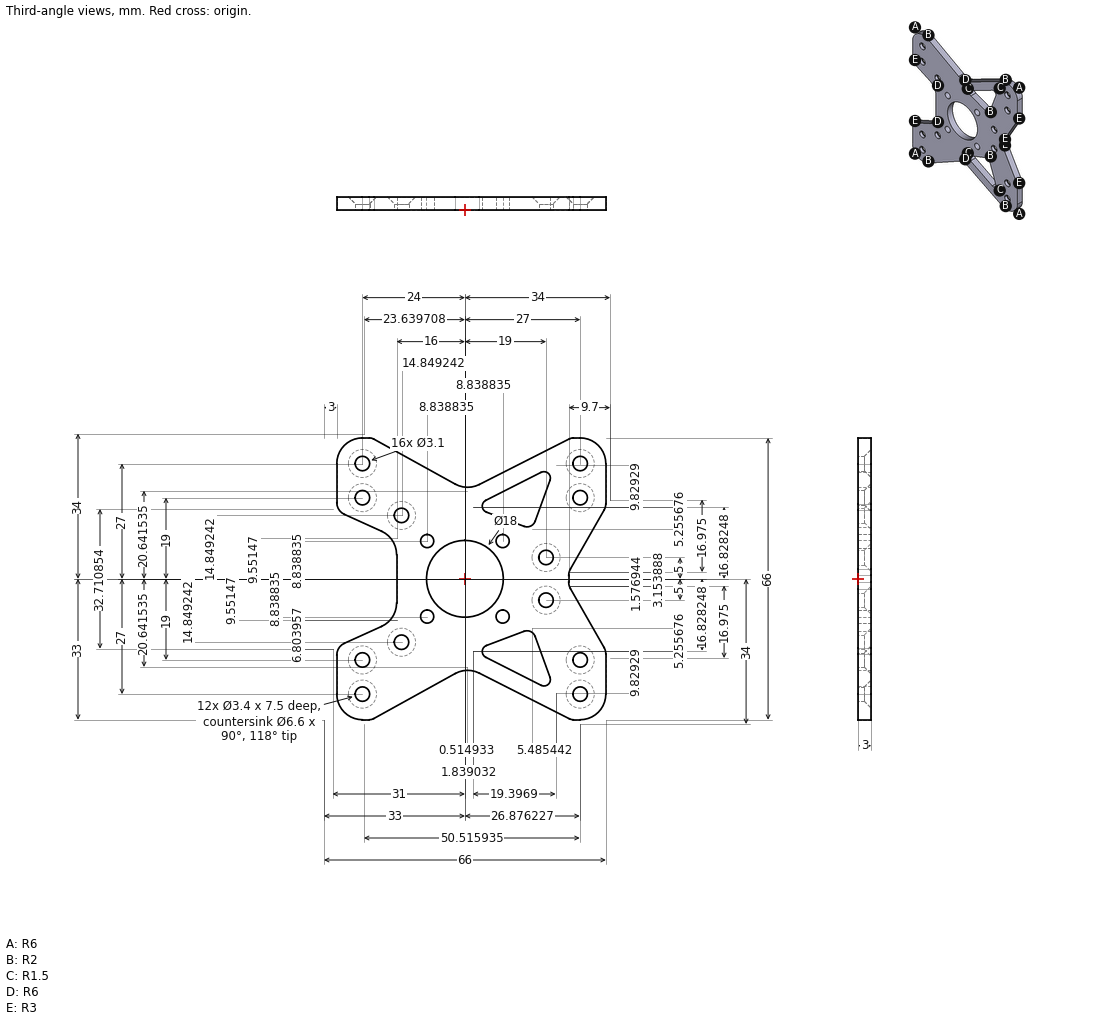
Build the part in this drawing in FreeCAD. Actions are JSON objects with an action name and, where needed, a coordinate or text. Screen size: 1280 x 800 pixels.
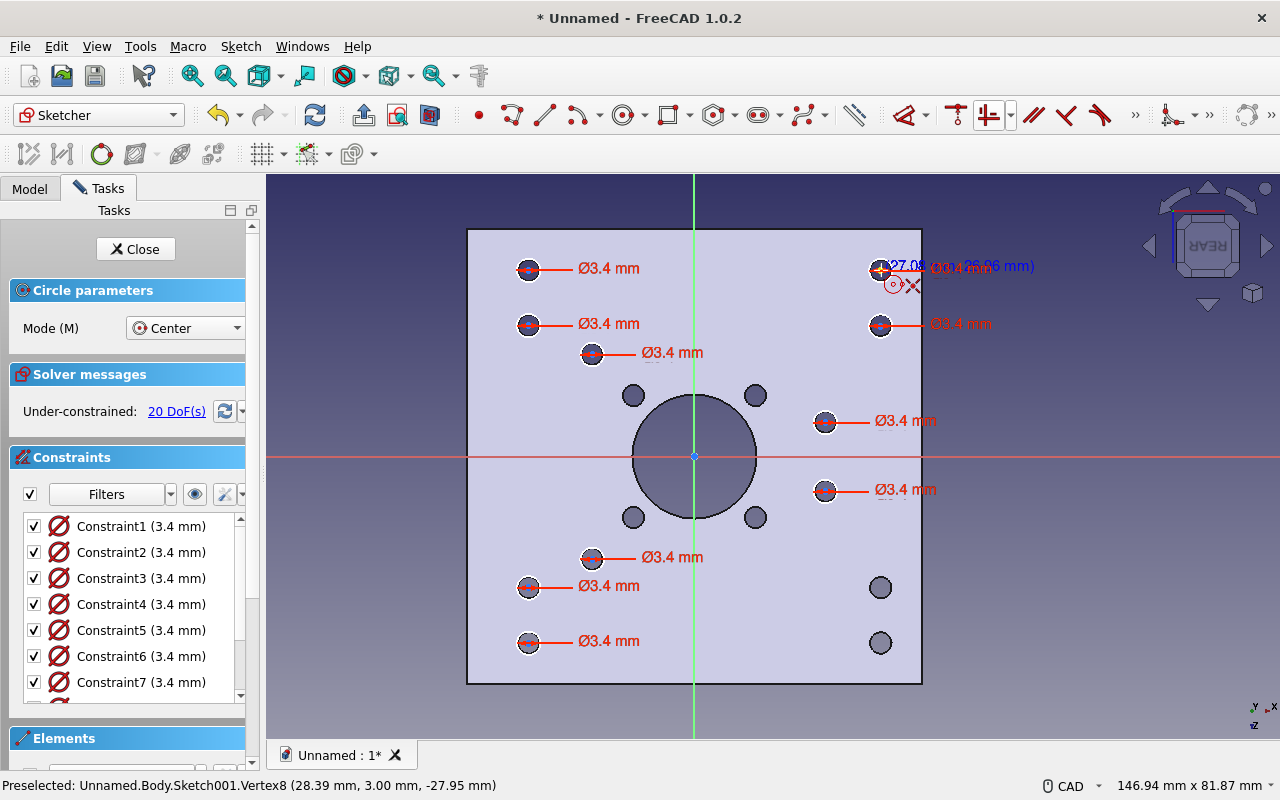
{"action": "scroll", "coordinate": [881, 588], "scroll_direction": "up", "scroll_amount": 4}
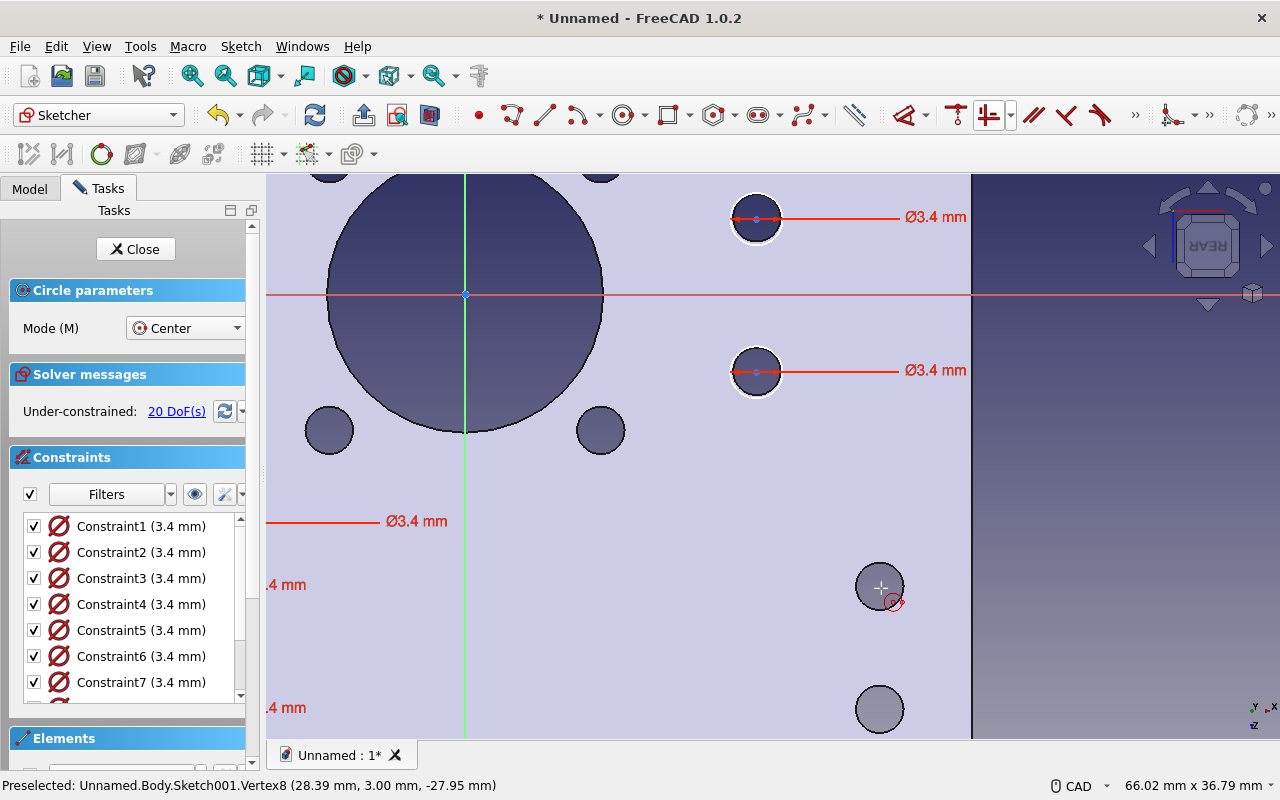
{"action": "left_click", "coordinate": [880, 586]}
{"action": "mouse_move", "coordinate": [898, 568]}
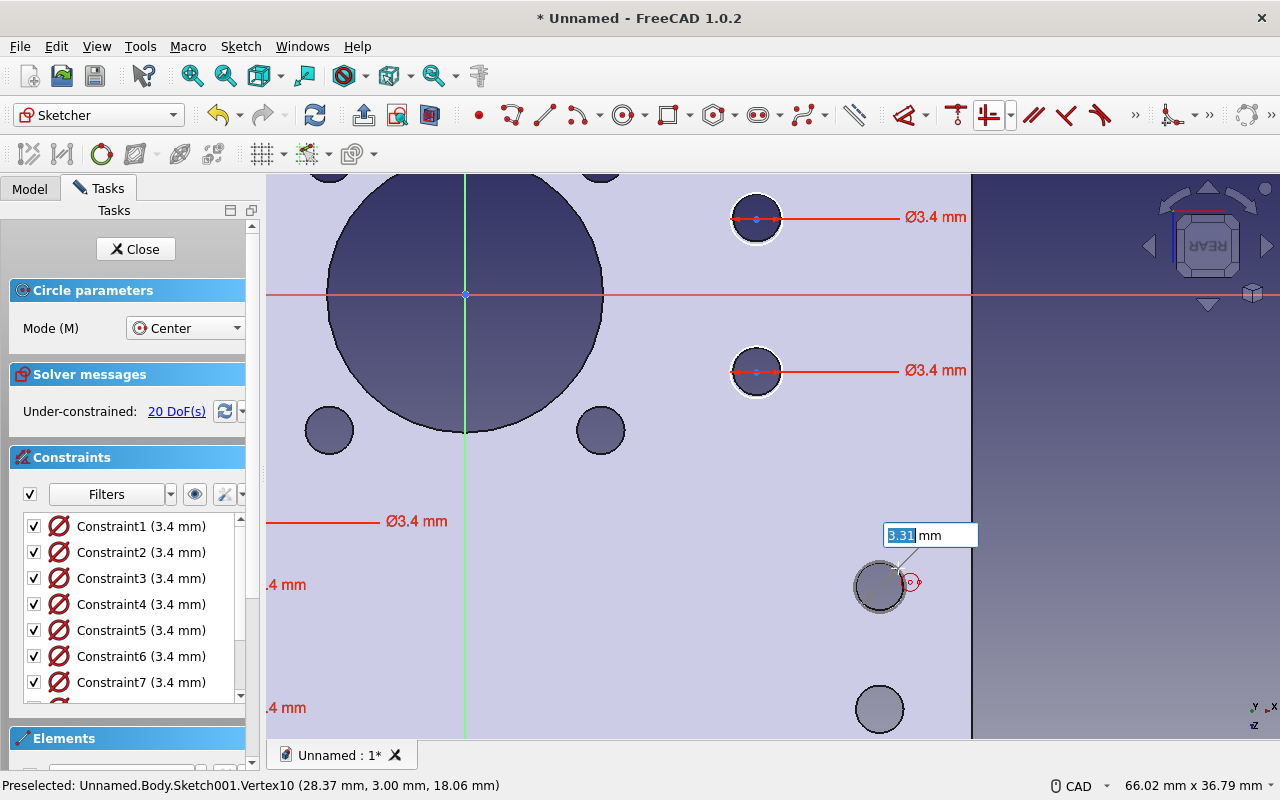
{"action": "type", "text": "3.4"}
{"action": "key", "text": "Return"}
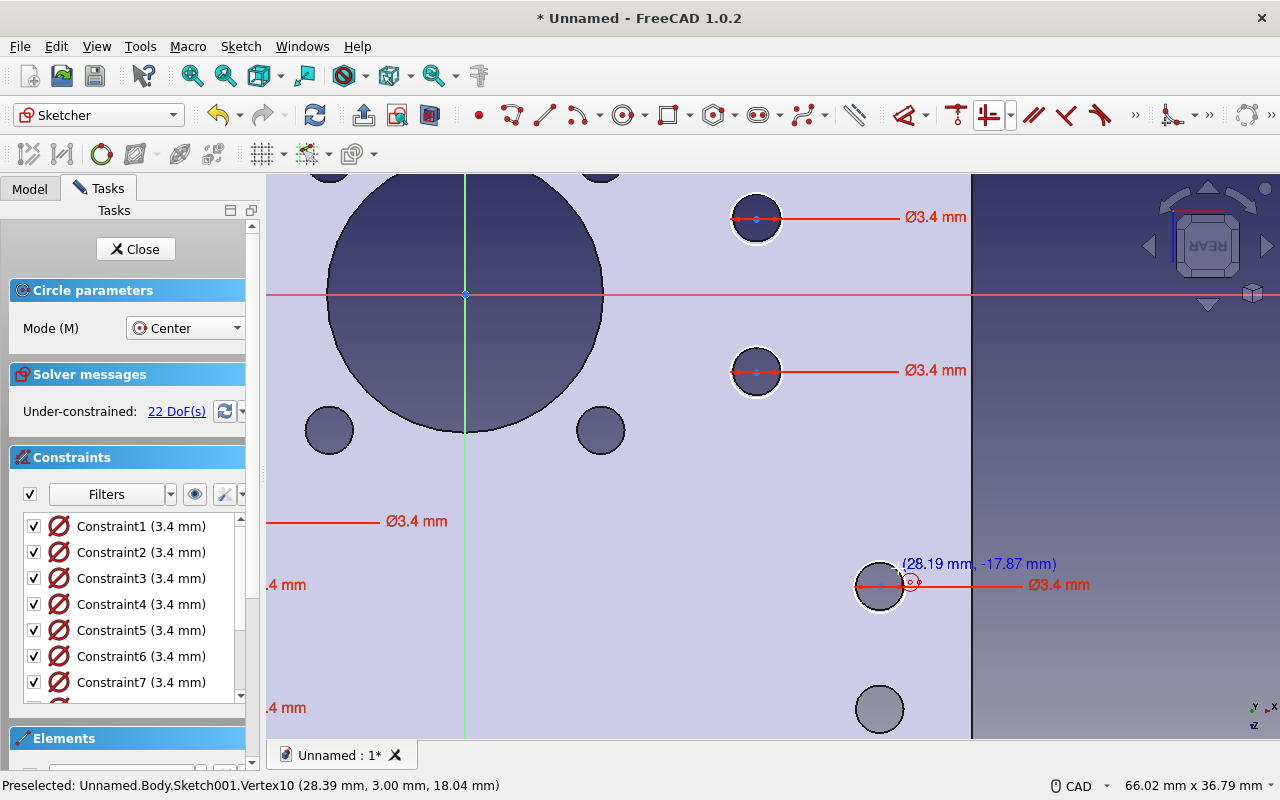
{"action": "left_click", "coordinate": [880, 709]}
{"action": "mouse_move", "coordinate": [898, 691]}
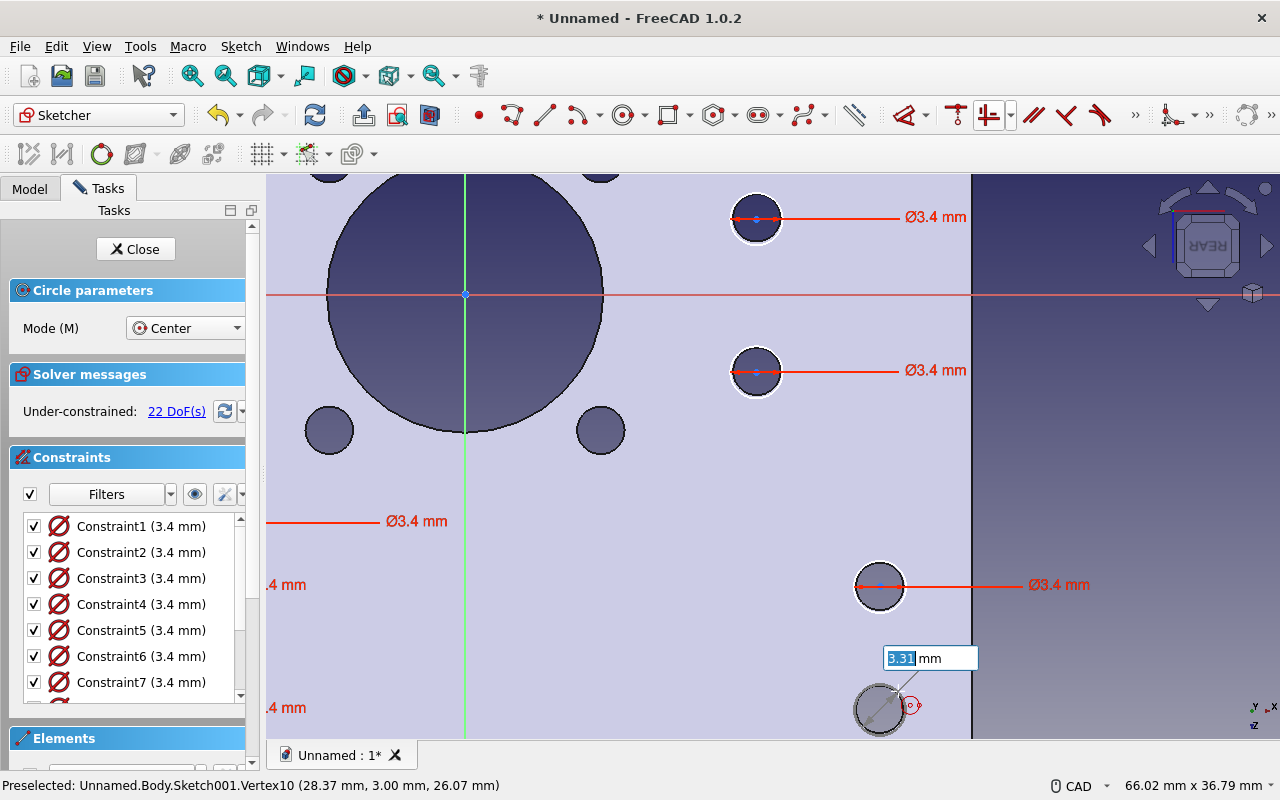
{"action": "type", "text": "3.4"}
{"action": "key", "text": "Return"}
{"action": "key", "text": "Escape"}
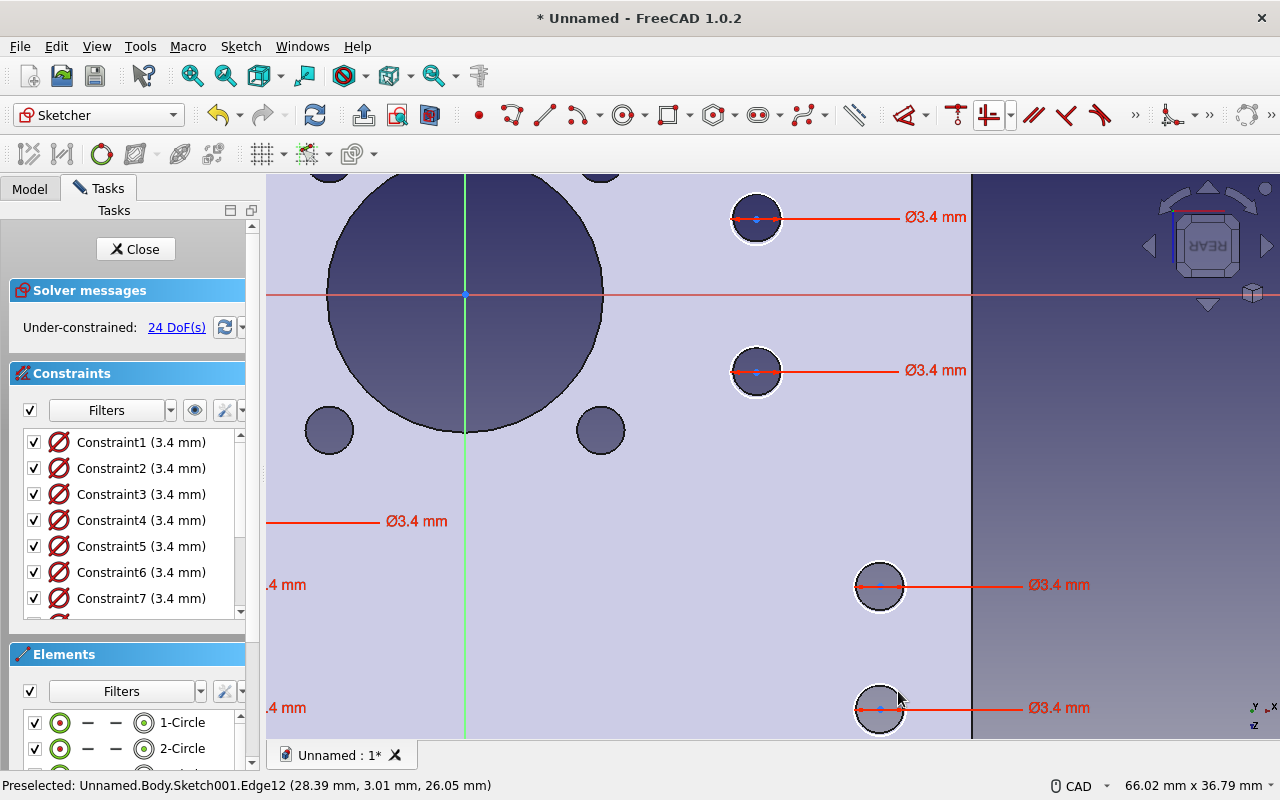
{"action": "scroll", "coordinate": [881, 589], "scroll_direction": "down", "scroll_amount": 4}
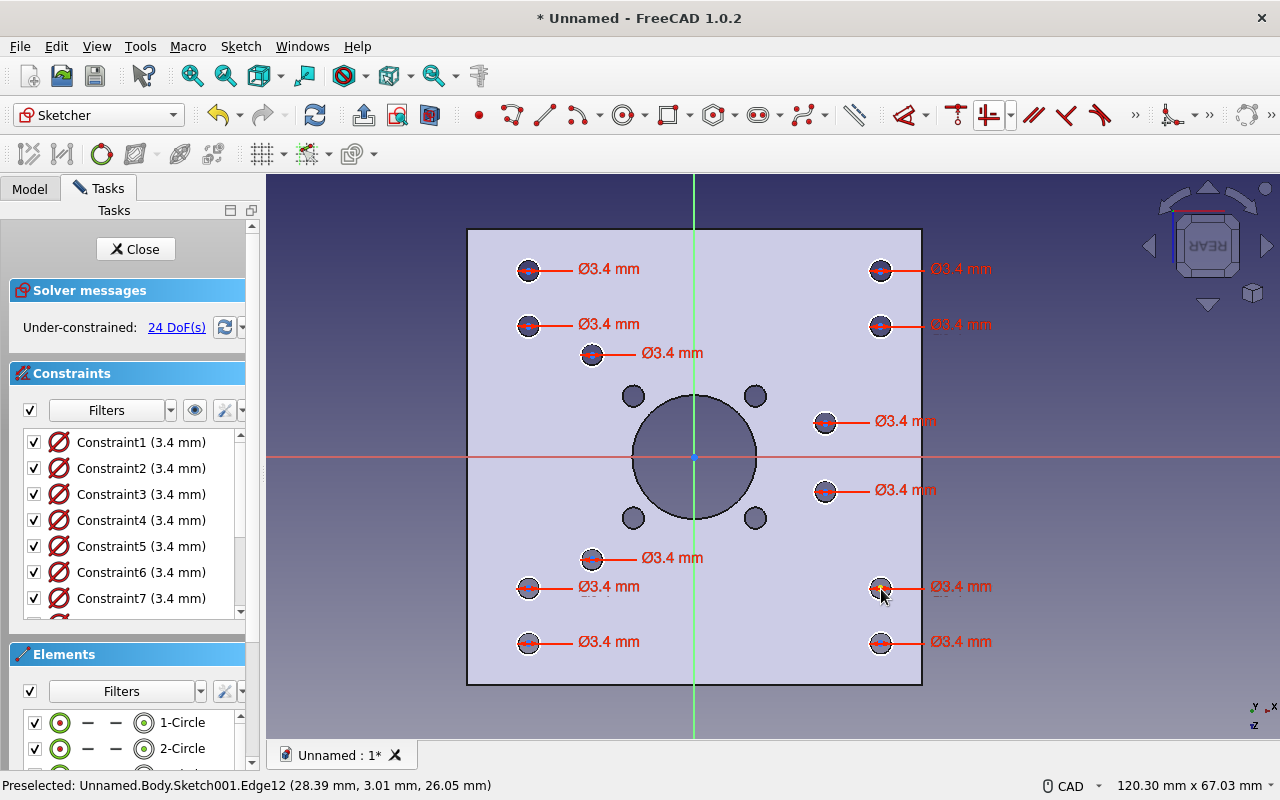
{"action": "left_click", "coordinate": [529, 271]}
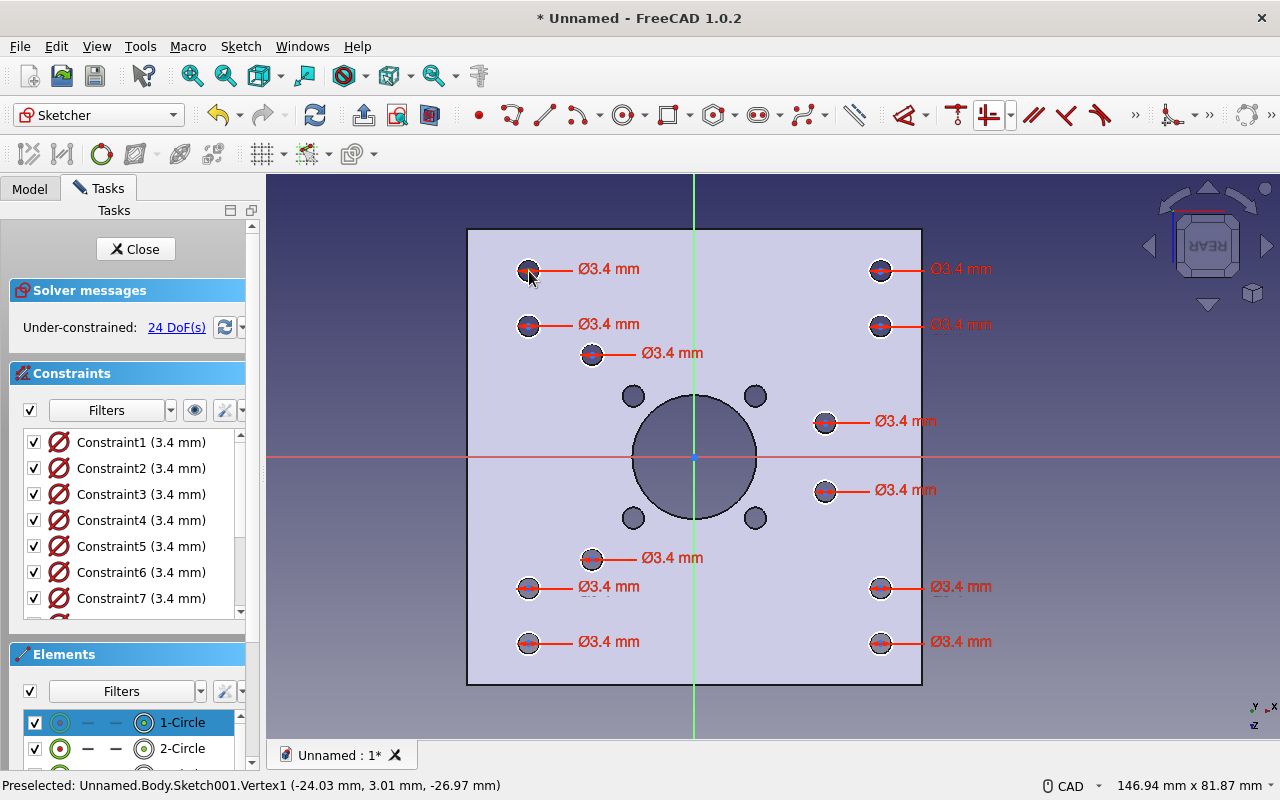
{"action": "left_click", "coordinate": [529, 326]}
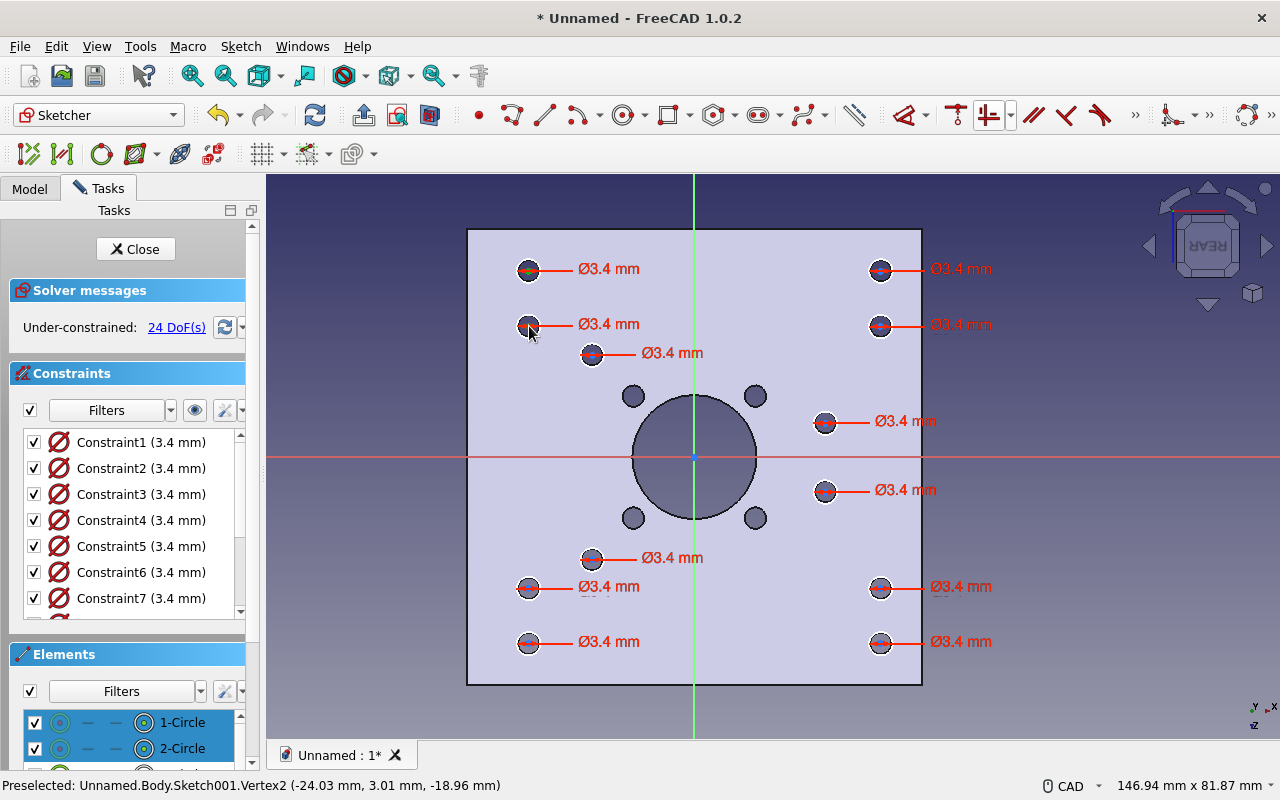
{"action": "key", "text": "v"}